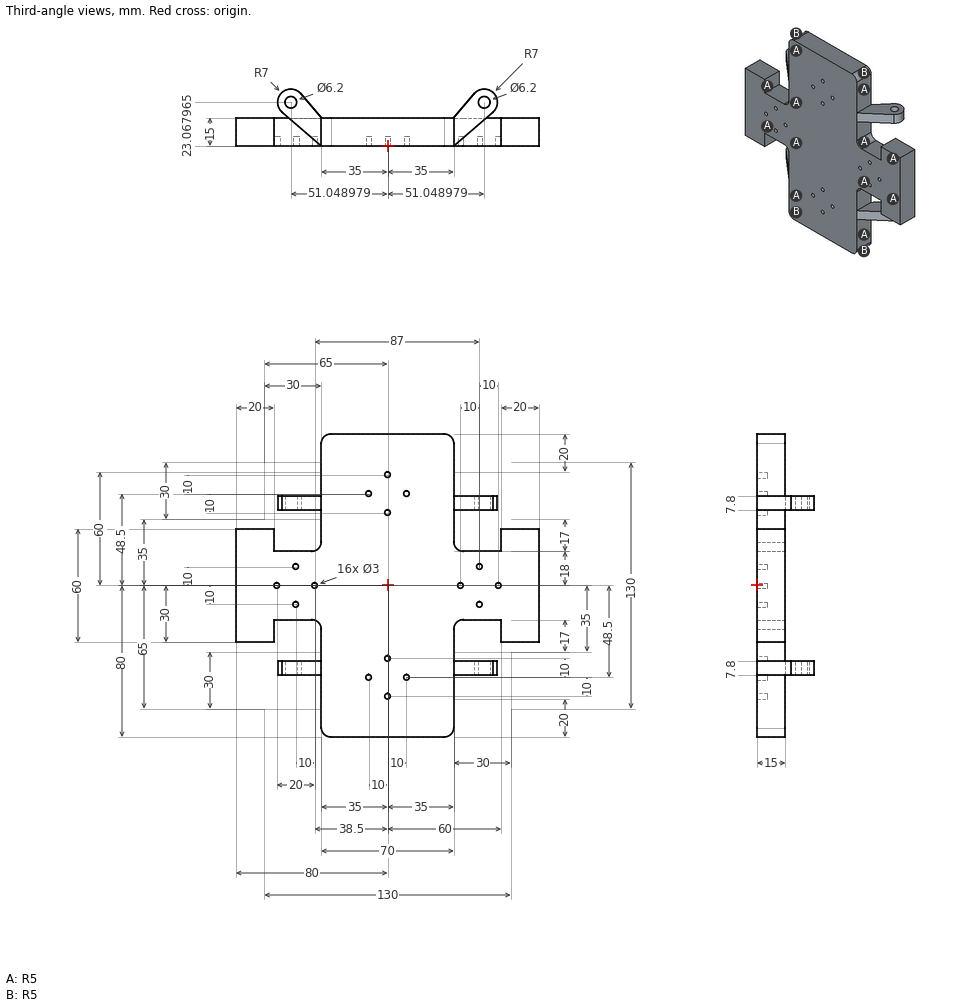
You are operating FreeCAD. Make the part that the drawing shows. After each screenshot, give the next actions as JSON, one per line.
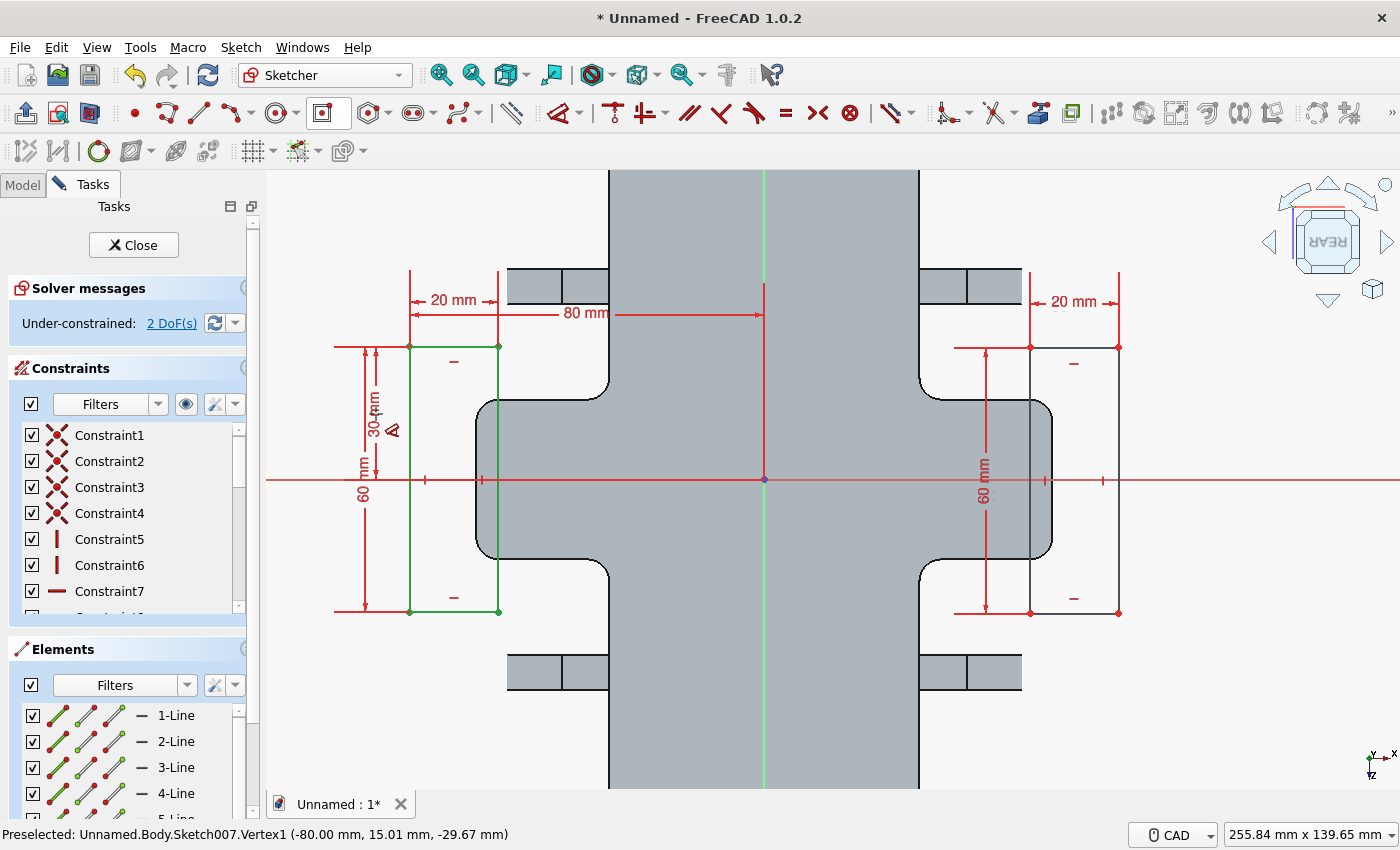
{"action": "left_click", "coordinate": [1030, 348]}
{"action": "left_click", "coordinate": [897, 314]}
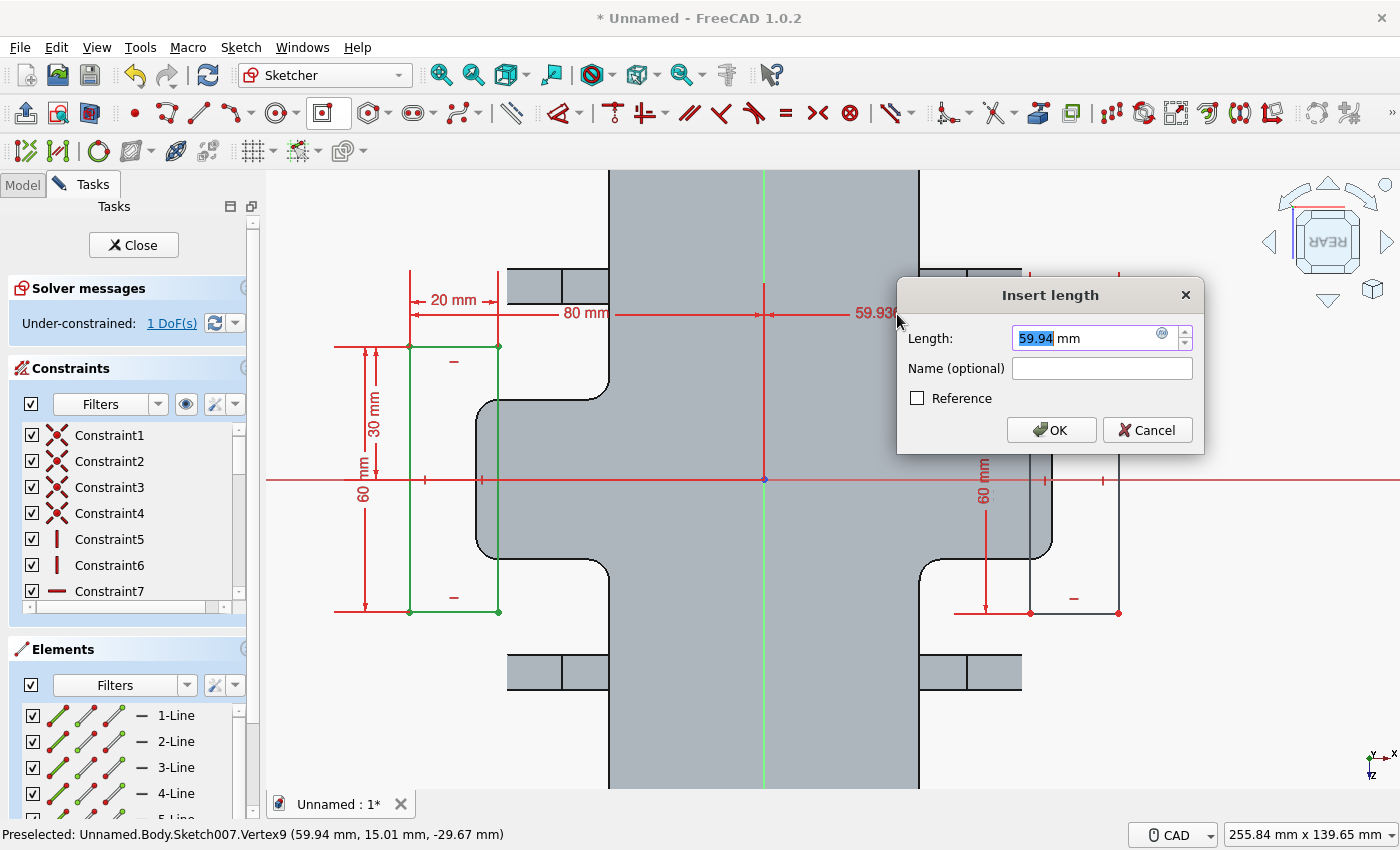
{"action": "type", "text": "60"}
{"action": "key", "text": "Return"}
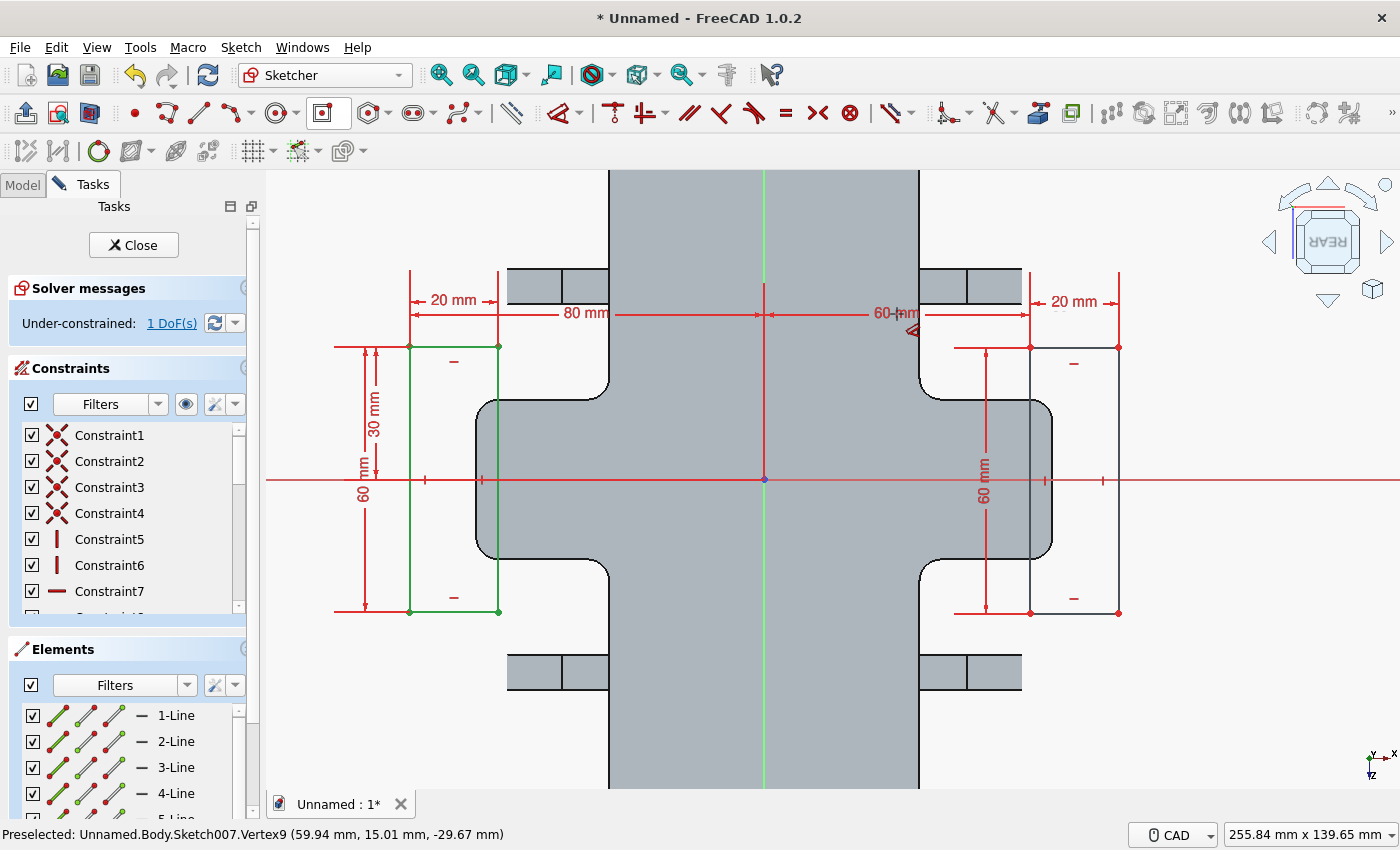
{"action": "left_click", "coordinate": [1030, 348]}
{"action": "left_click", "coordinate": [1064, 414]}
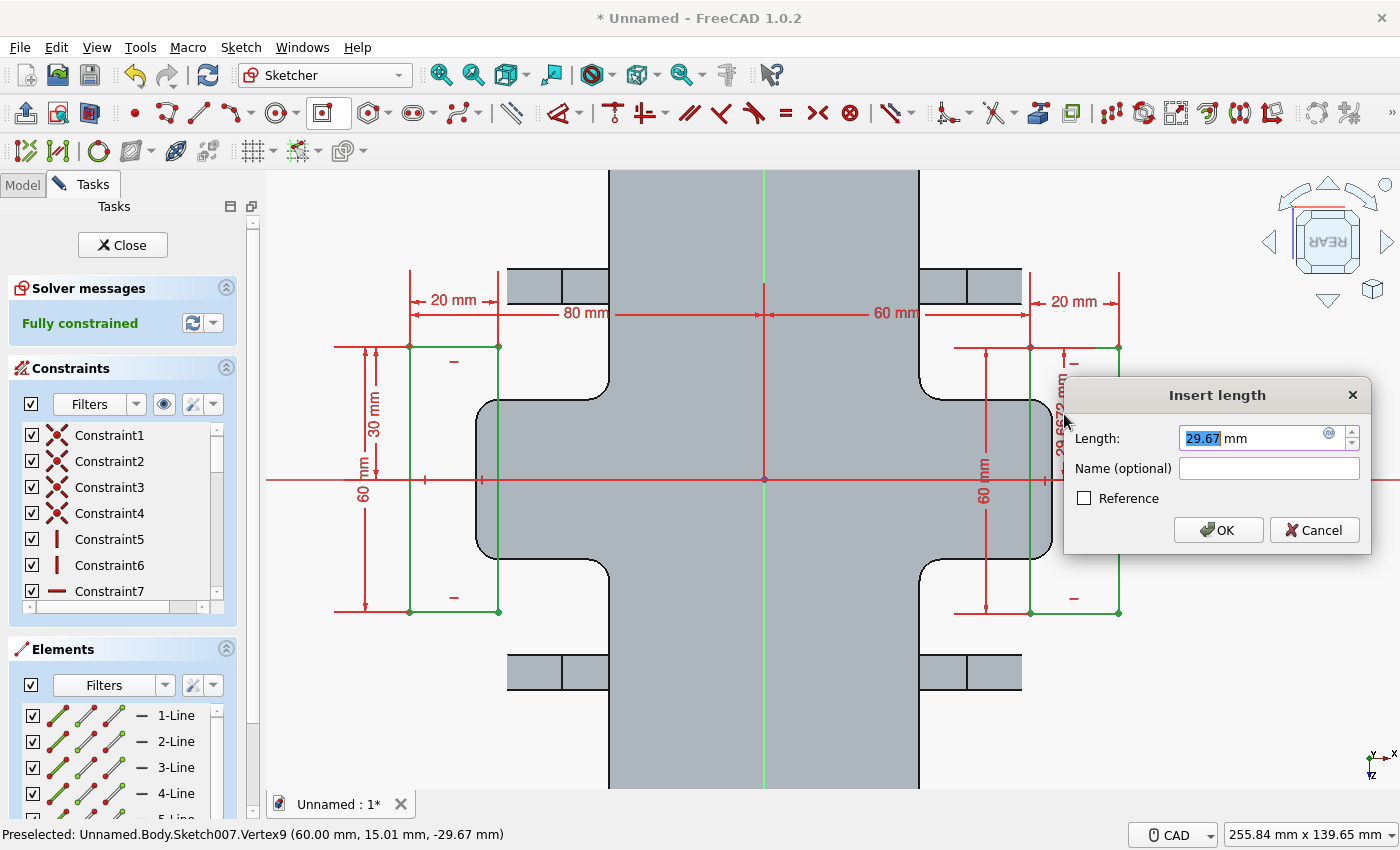
{"action": "type", "text": "30"}
{"action": "key", "text": "Return"}
{"action": "key", "text": "Escape"}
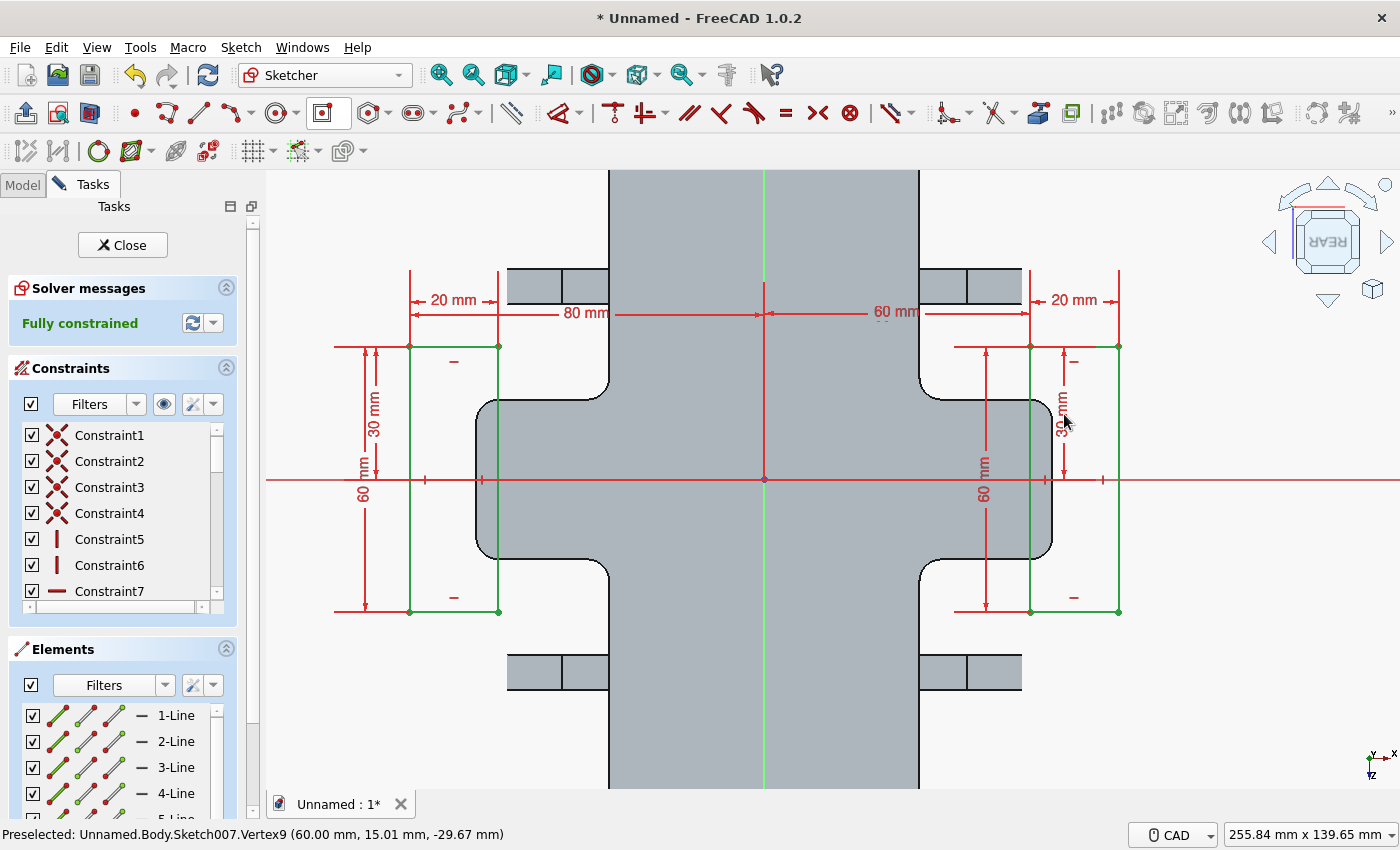
{"action": "left_click", "coordinate": [123, 245]}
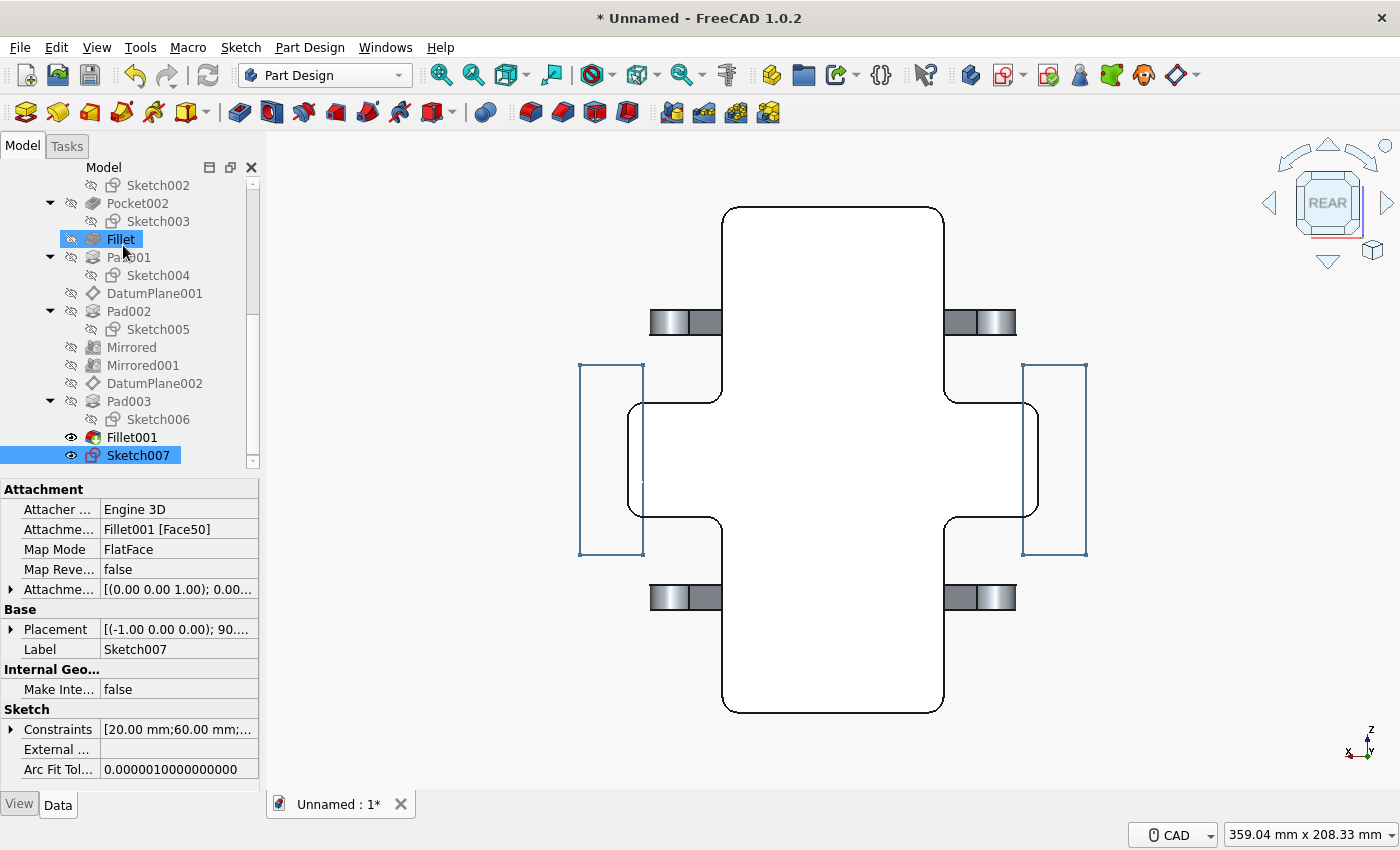
{"action": "left_click", "coordinate": [26, 112]}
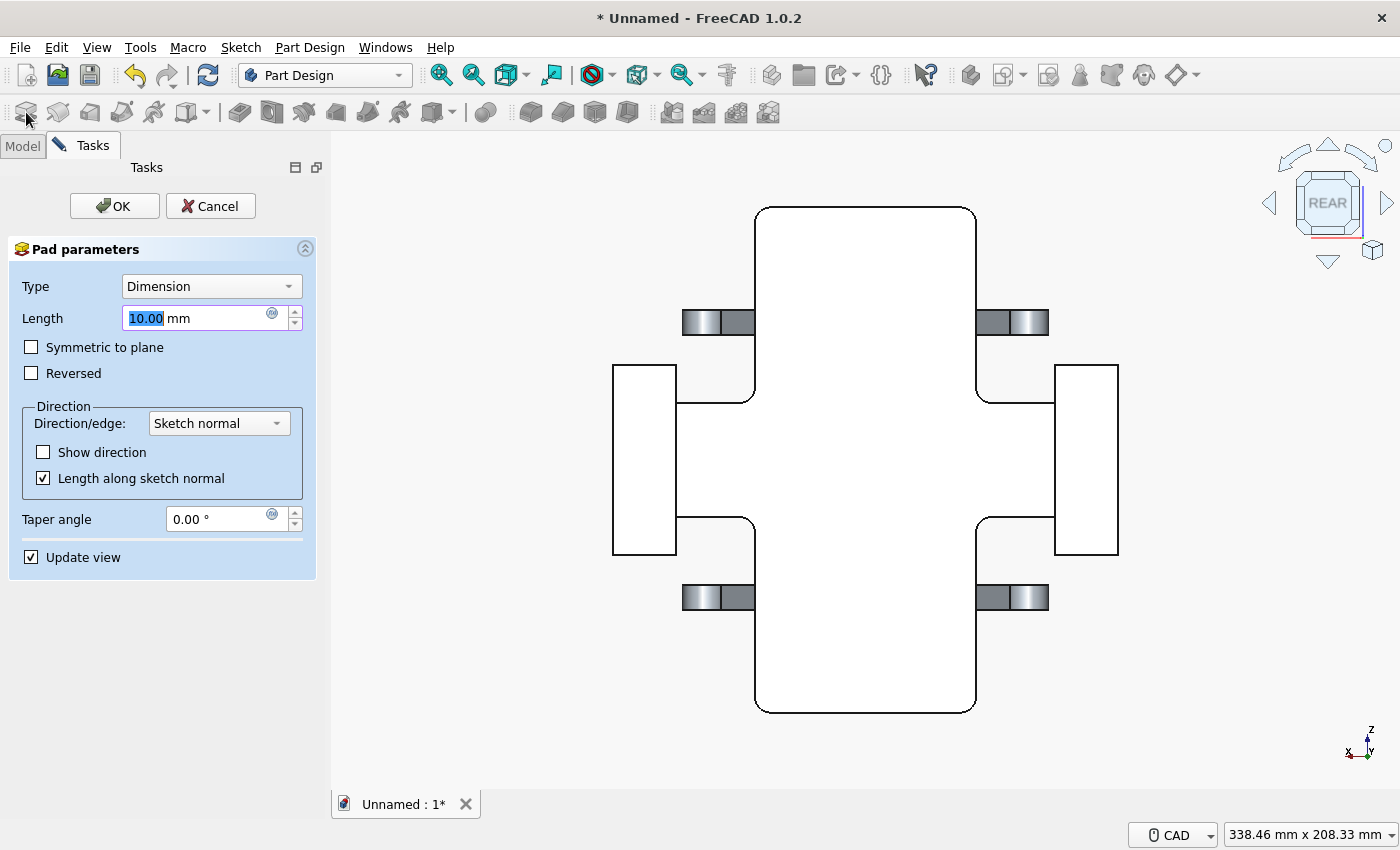
{"action": "type", "text": "15"}
{"action": "key", "text": "Tab"}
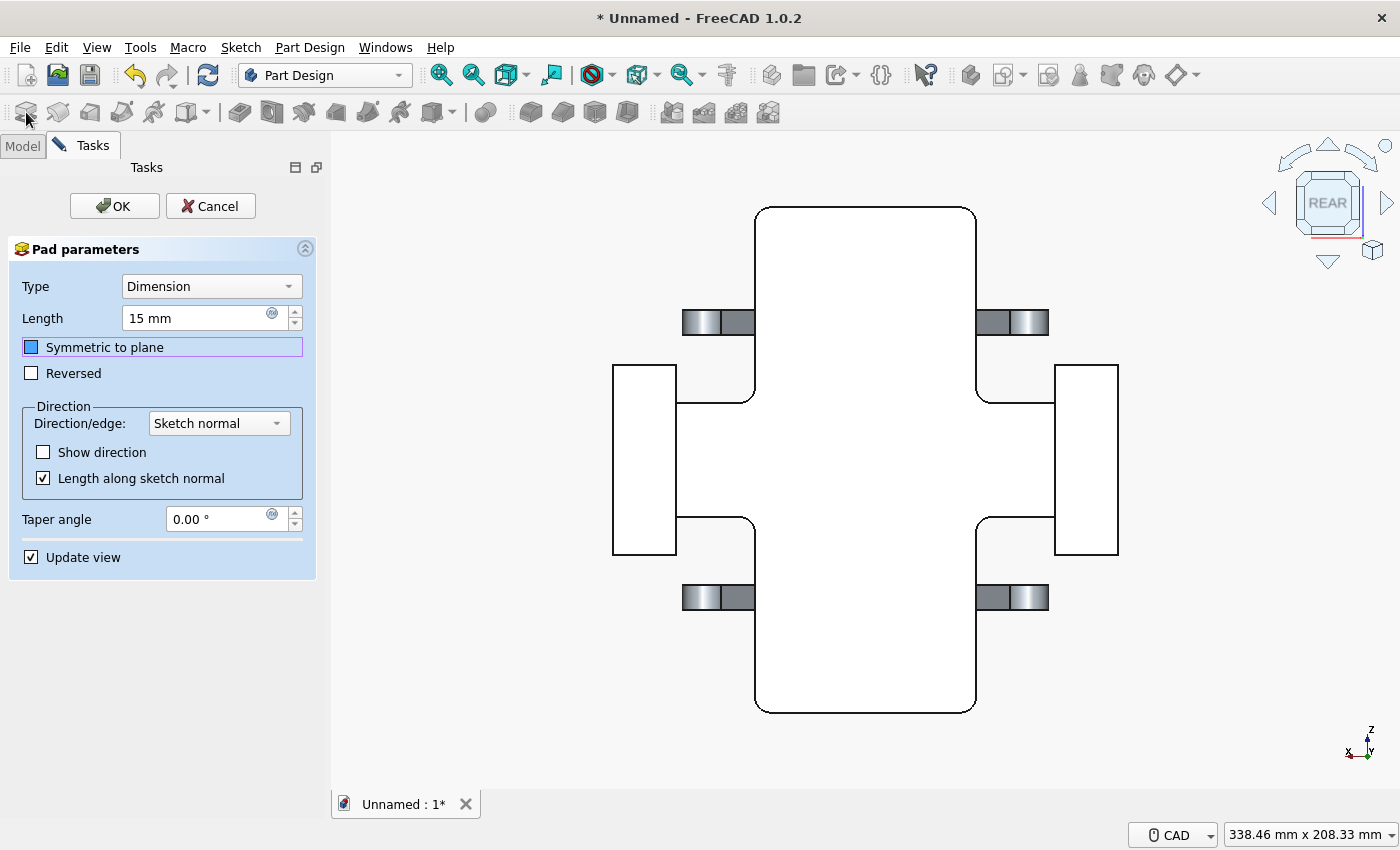
{"action": "left_click", "coordinate": [30, 373]}